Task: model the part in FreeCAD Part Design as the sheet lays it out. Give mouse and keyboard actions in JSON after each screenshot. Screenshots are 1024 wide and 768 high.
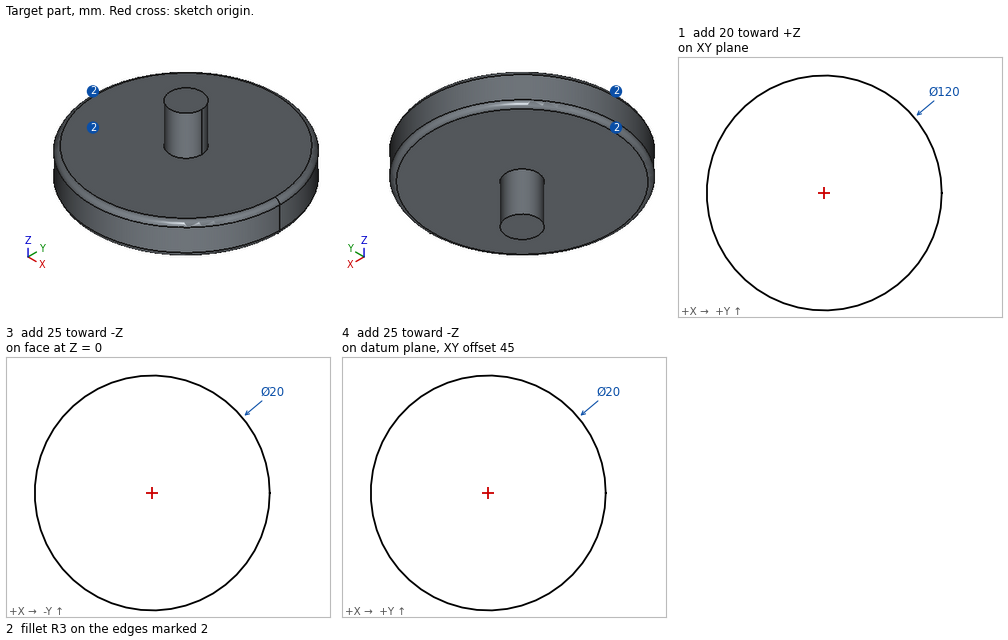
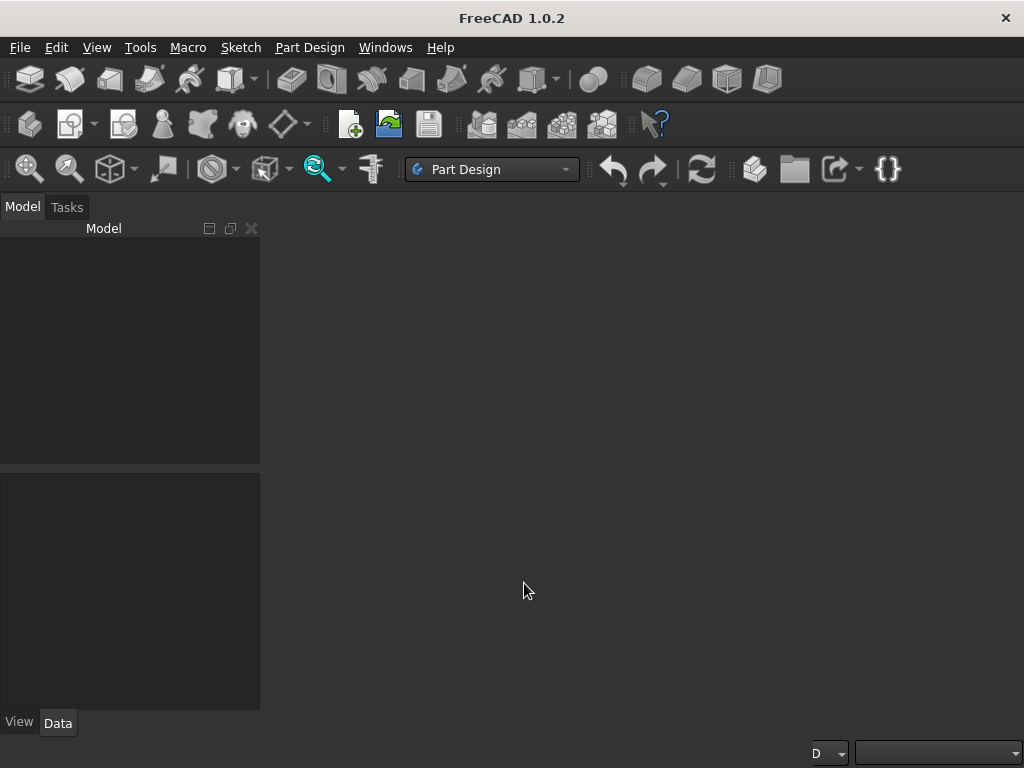
{"action": "key", "text": "ctrl+n"}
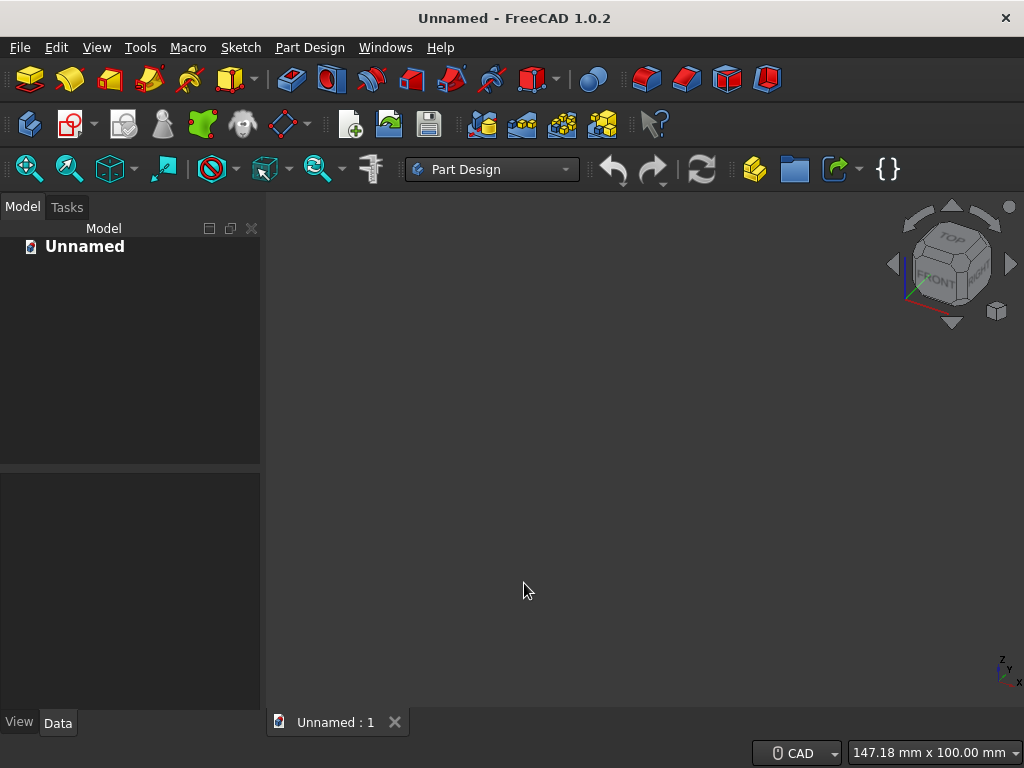
{"action": "left_click", "coordinate": [70, 124]}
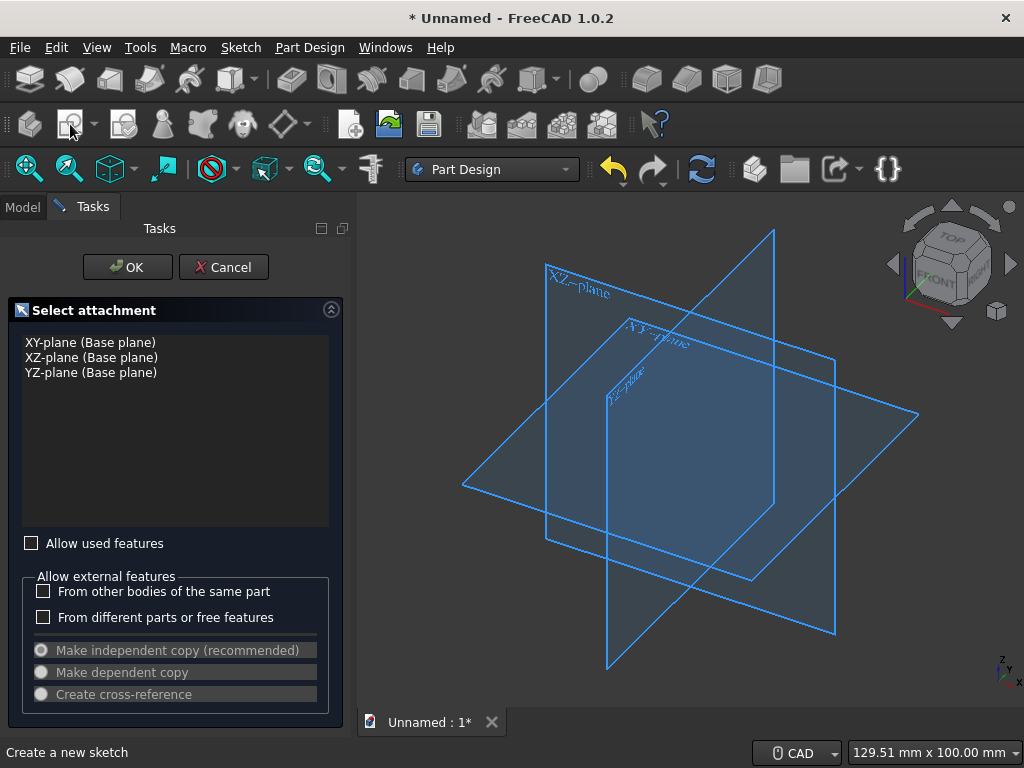
{"action": "left_click", "coordinate": [82, 342]}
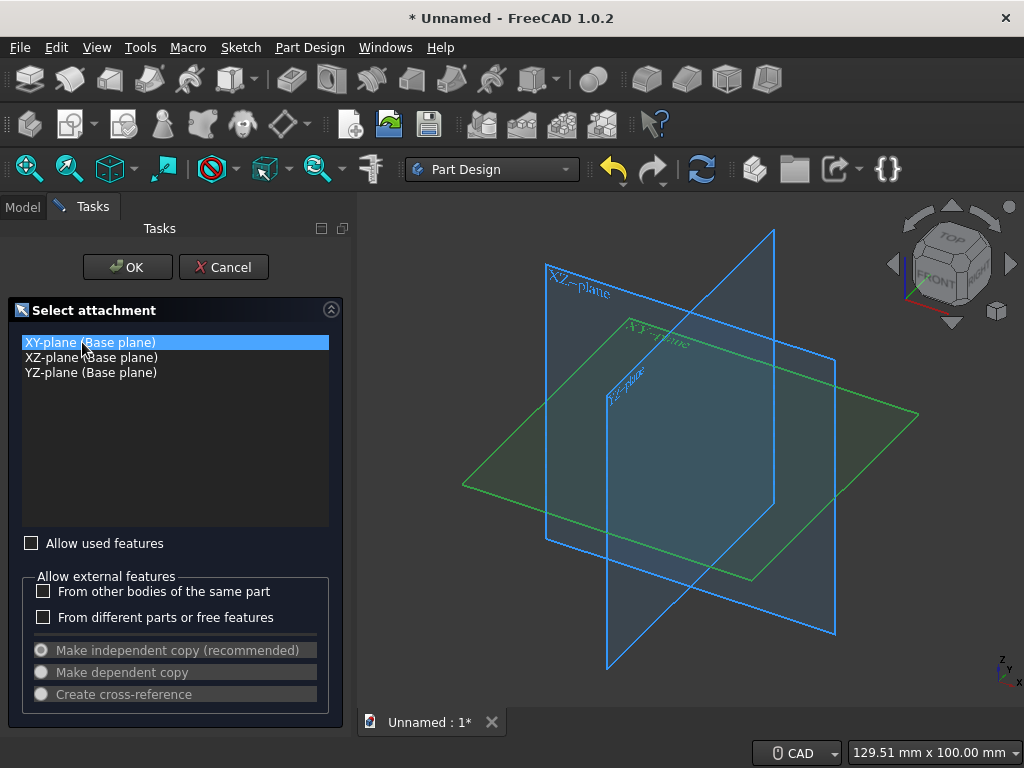
{"action": "left_click", "coordinate": [128, 267]}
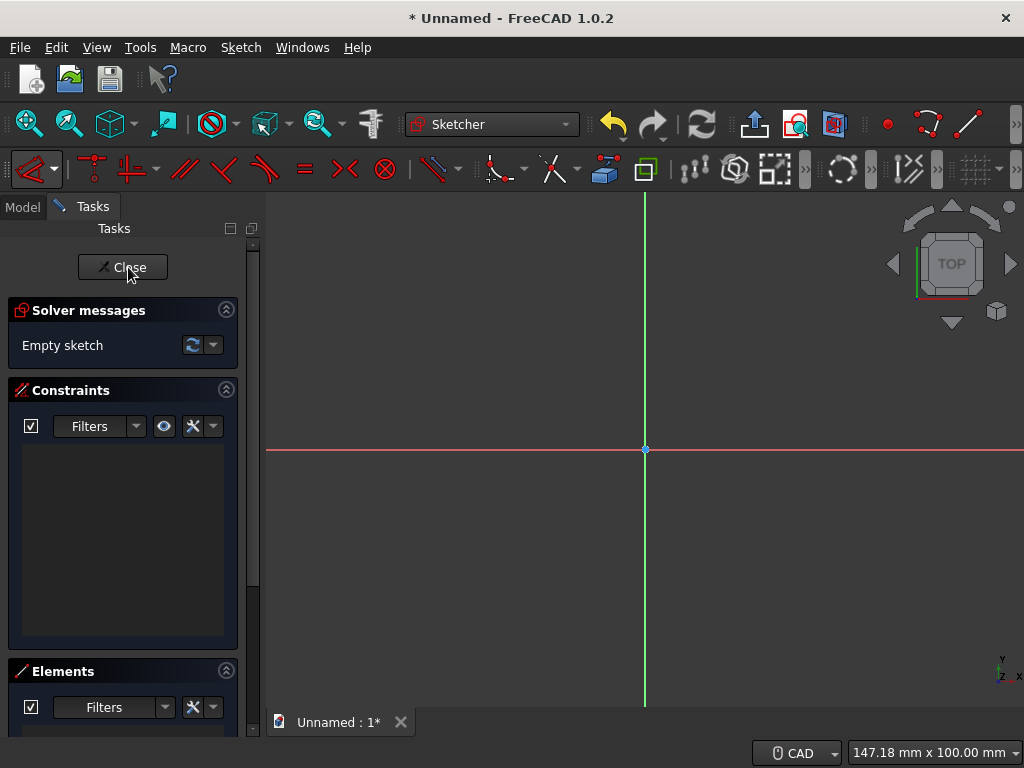
{"action": "scroll", "coordinate": [493, 450], "scroll_direction": "down", "scroll_amount": 3}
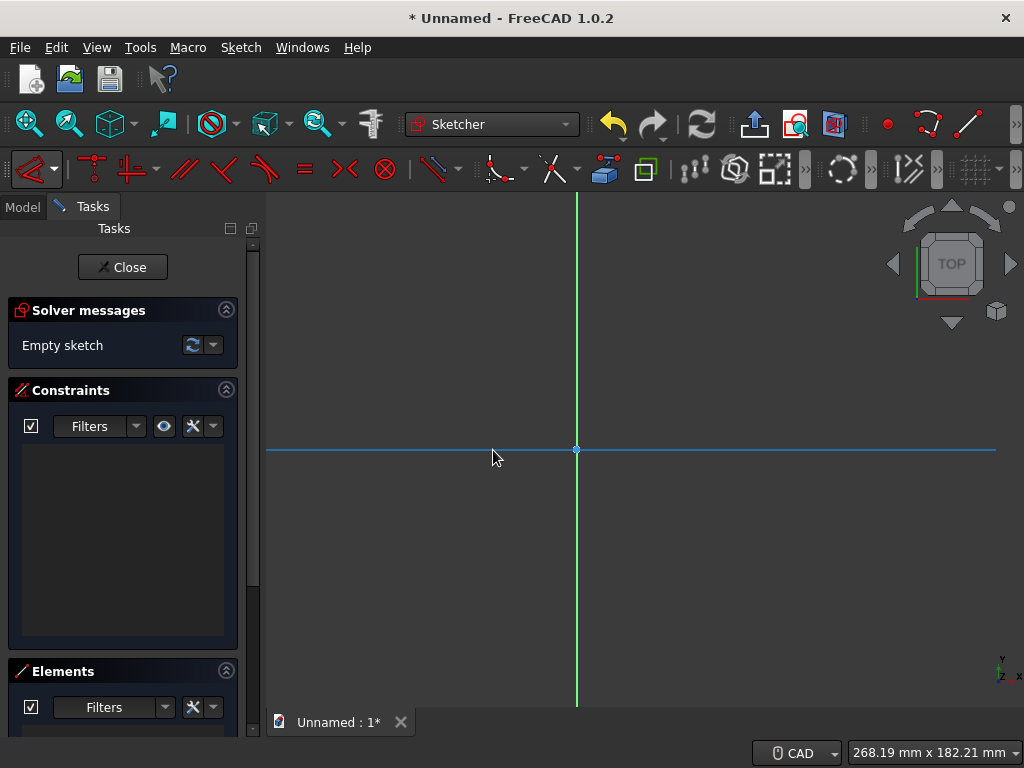
{"action": "key", "text": "g c"}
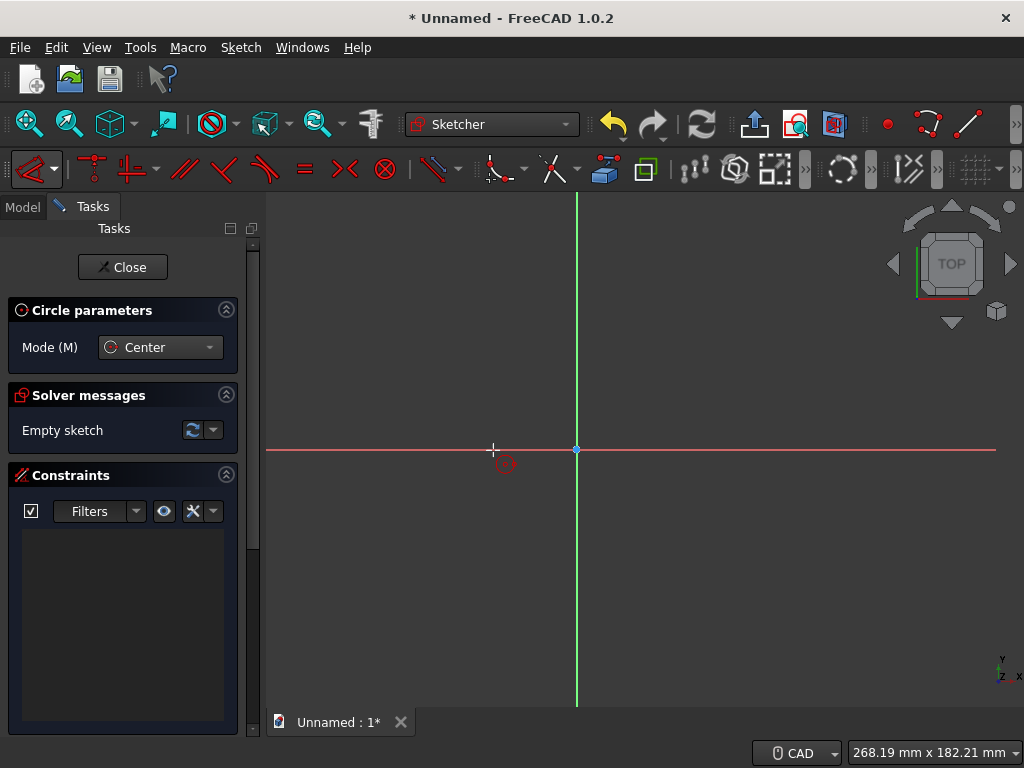
{"action": "left_click", "coordinate": [577, 450]}
{"action": "left_click", "coordinate": [696, 330]}
{"action": "key", "text": "Escape"}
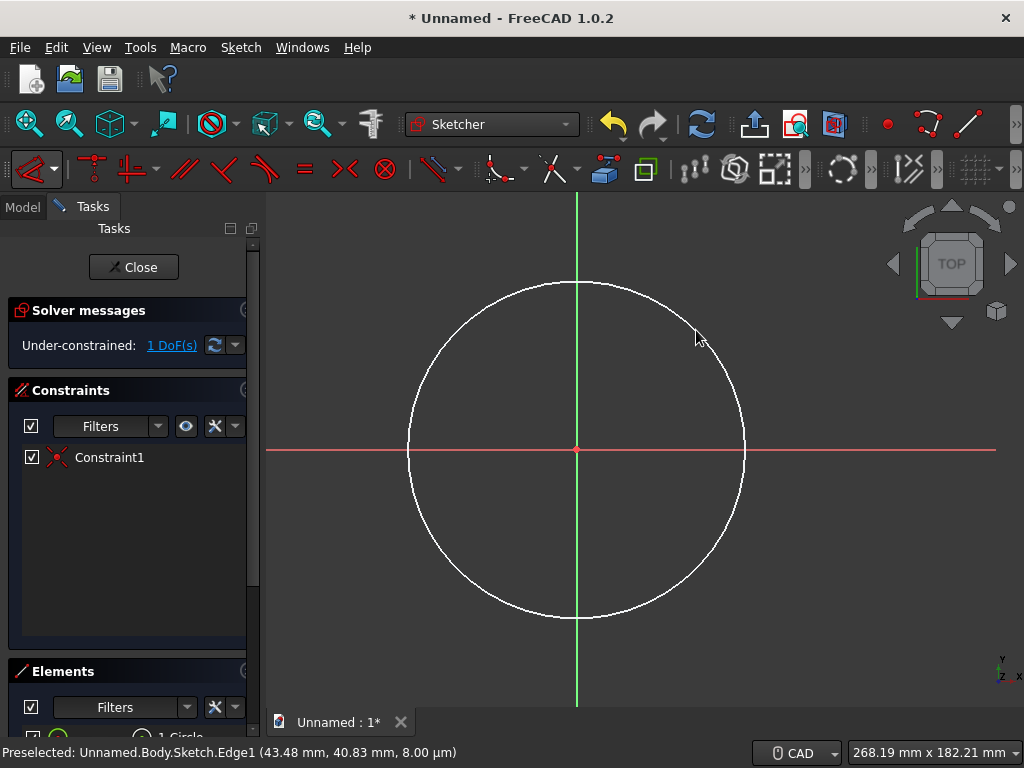
{"action": "left_click", "coordinate": [695, 330]}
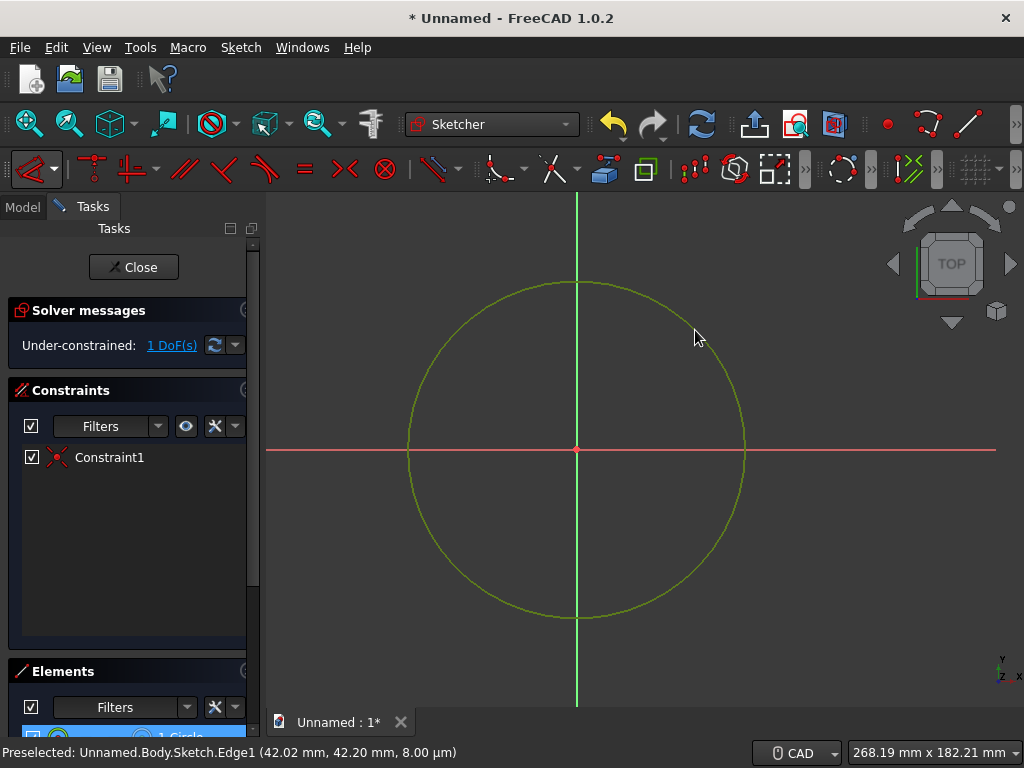
{"action": "key", "text": "k o"}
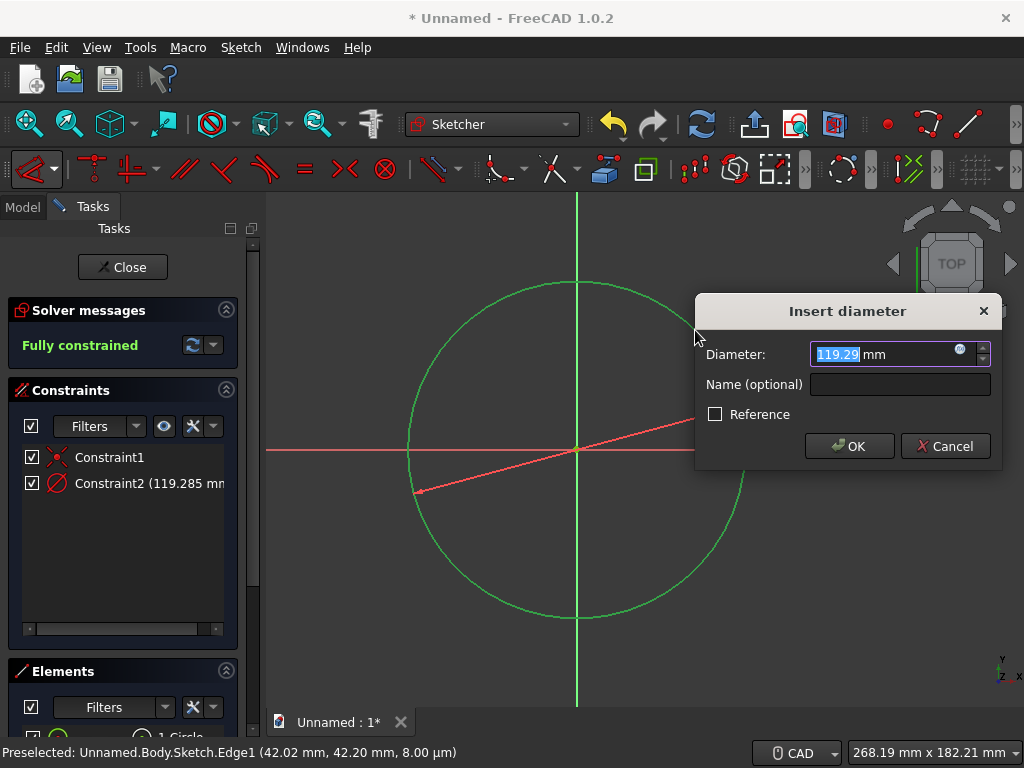
{"action": "type", "text": "120"}
{"action": "key", "text": "Return"}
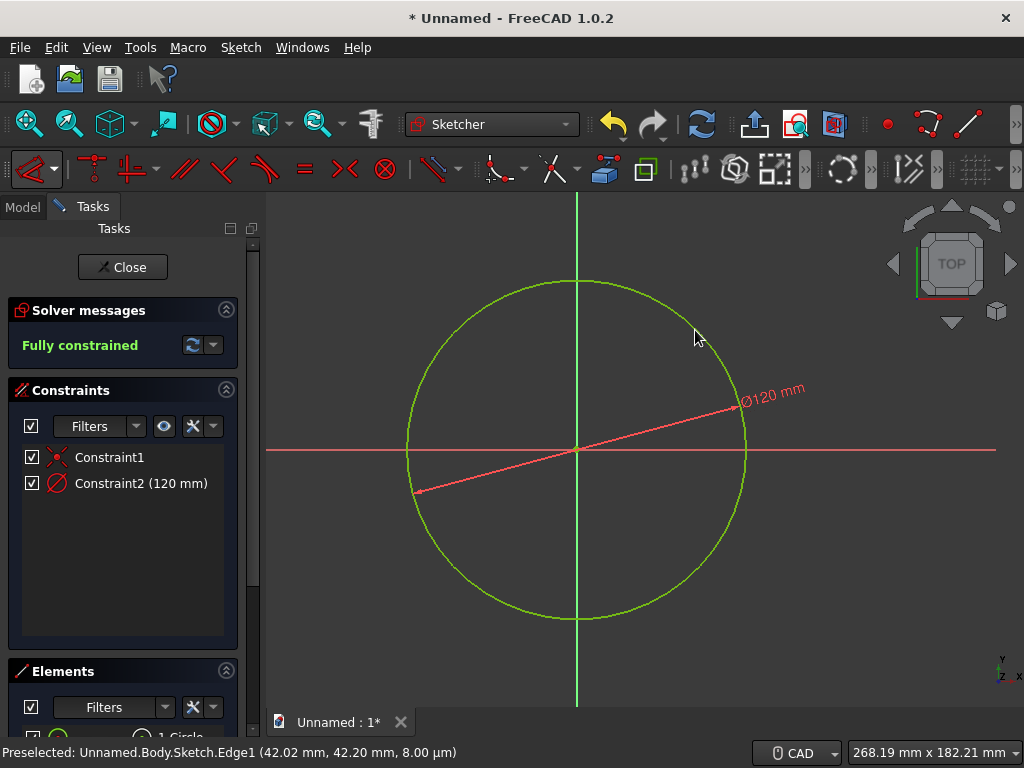
{"action": "left_click", "coordinate": [123, 267]}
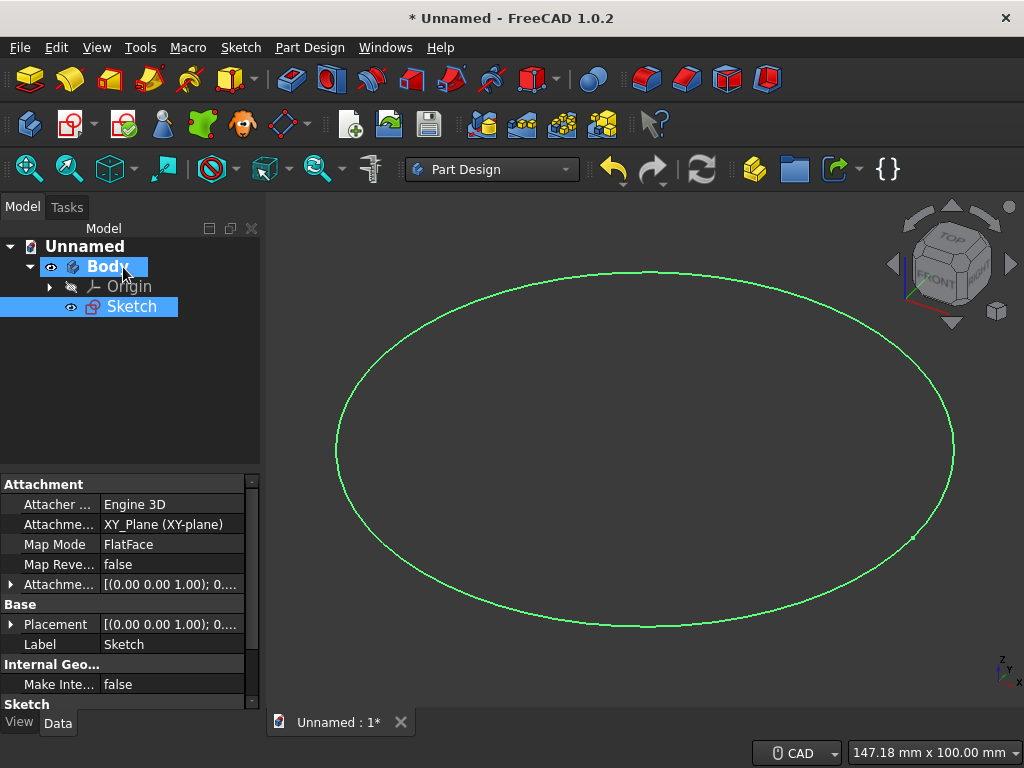
{"action": "left_click", "coordinate": [30, 80]}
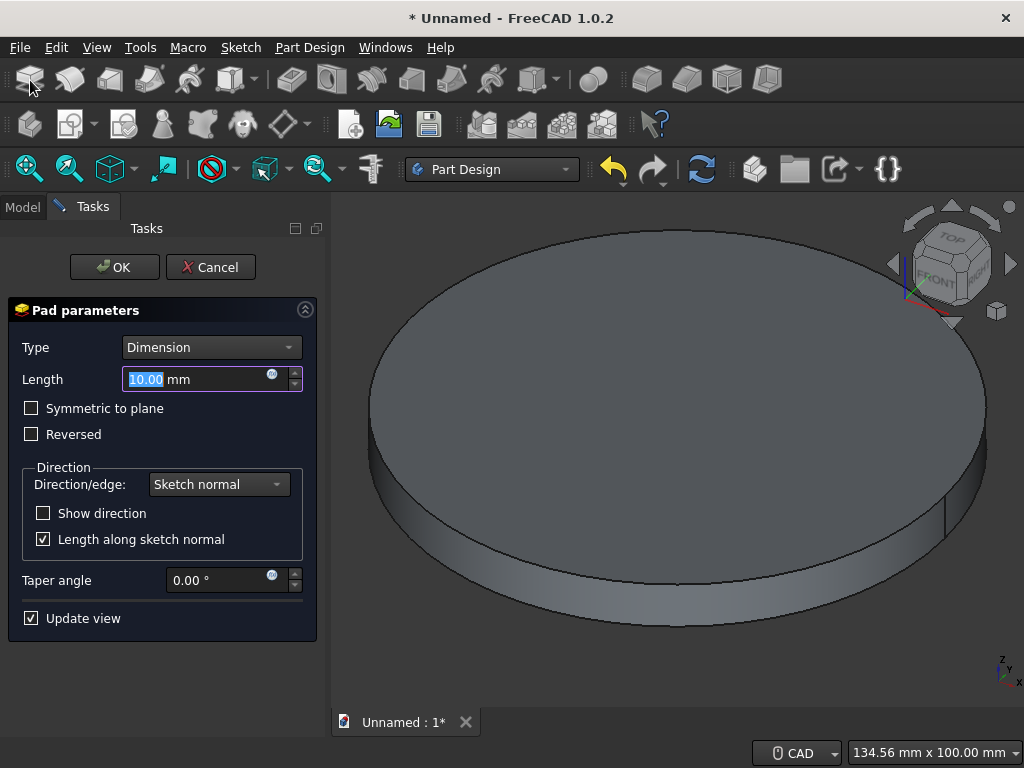
{"action": "type", "text": "20"}
{"action": "key", "text": "Tab"}